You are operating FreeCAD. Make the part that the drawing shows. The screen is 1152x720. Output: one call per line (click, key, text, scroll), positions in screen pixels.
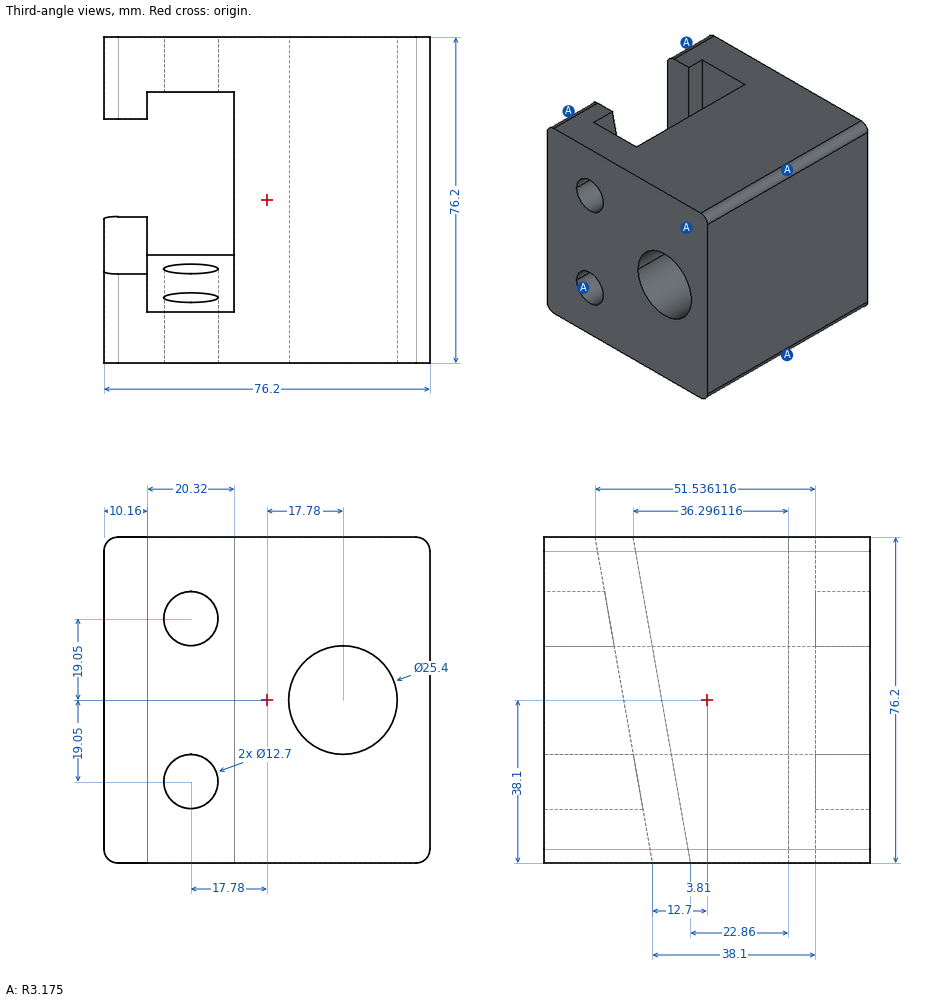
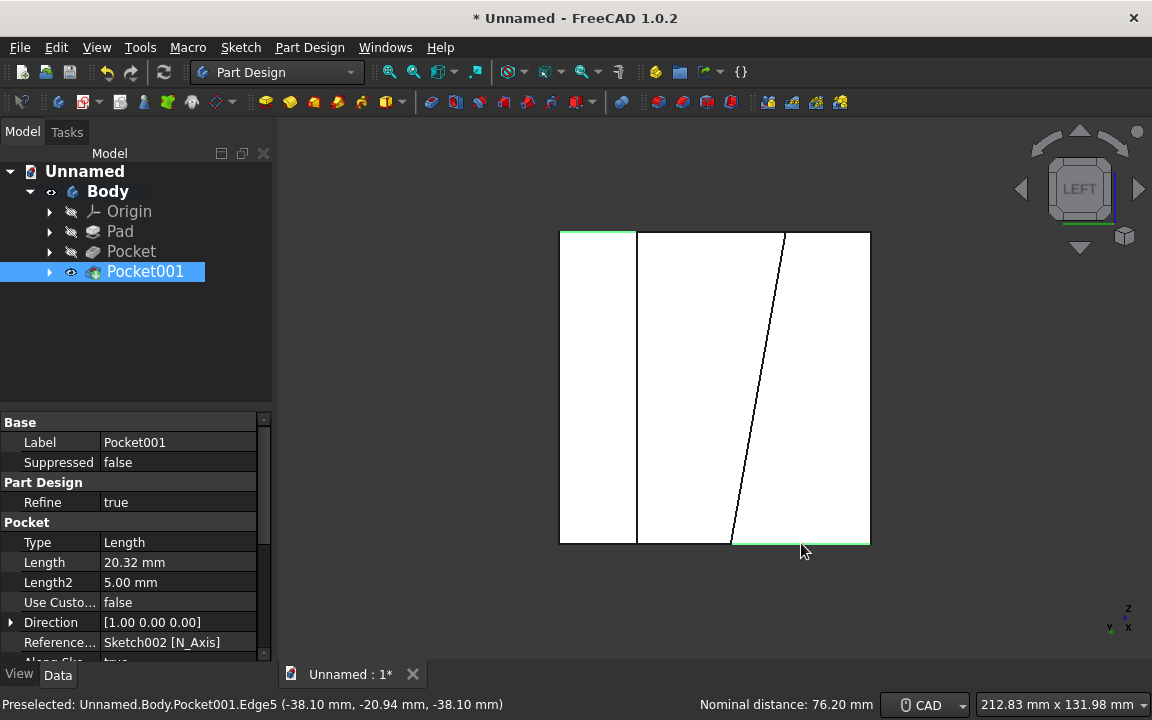
click(829, 231, ctrl)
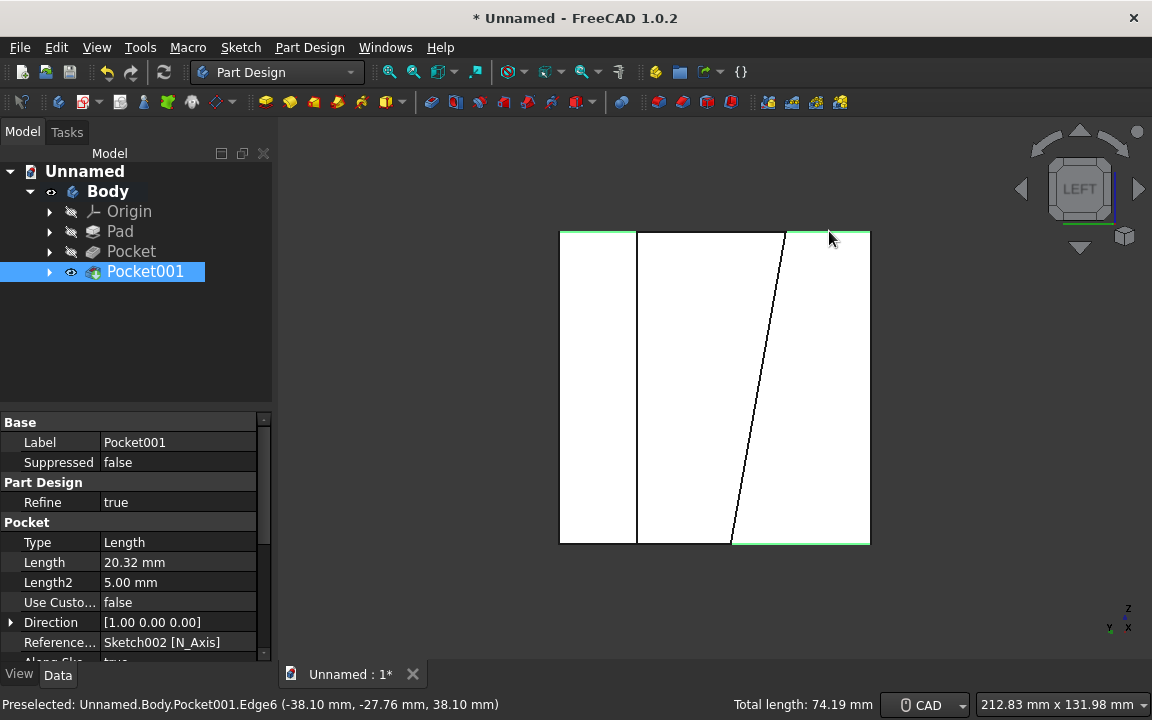
click(598, 543, ctrl)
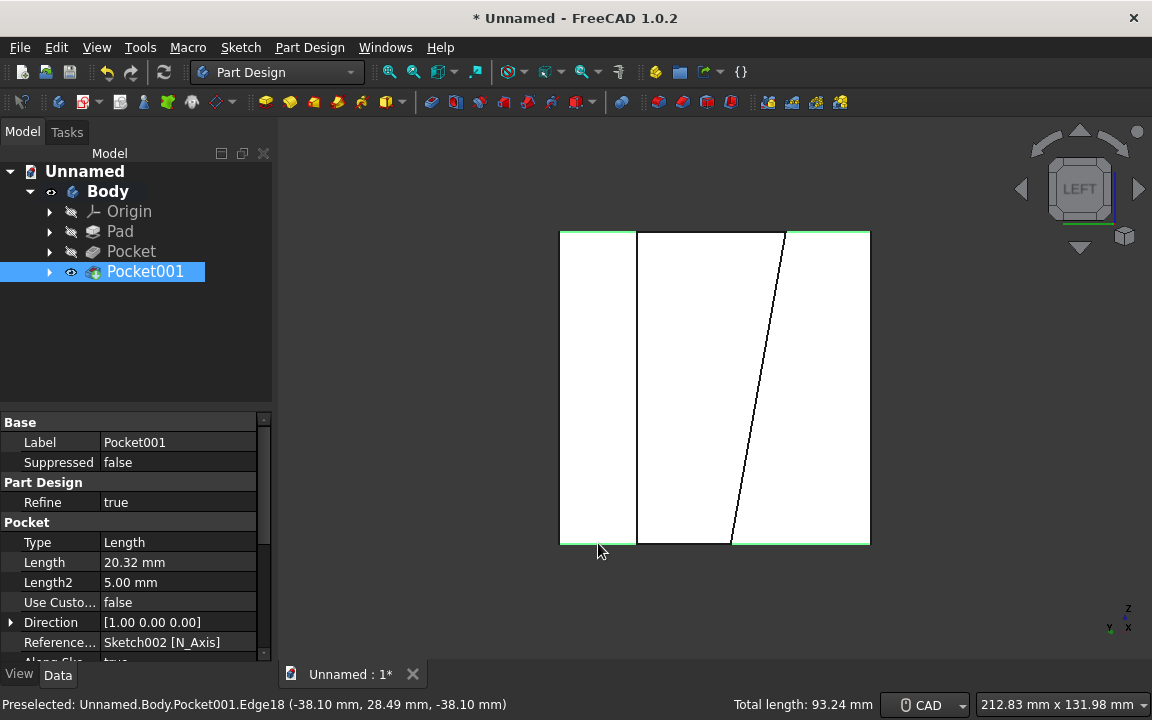
key(0)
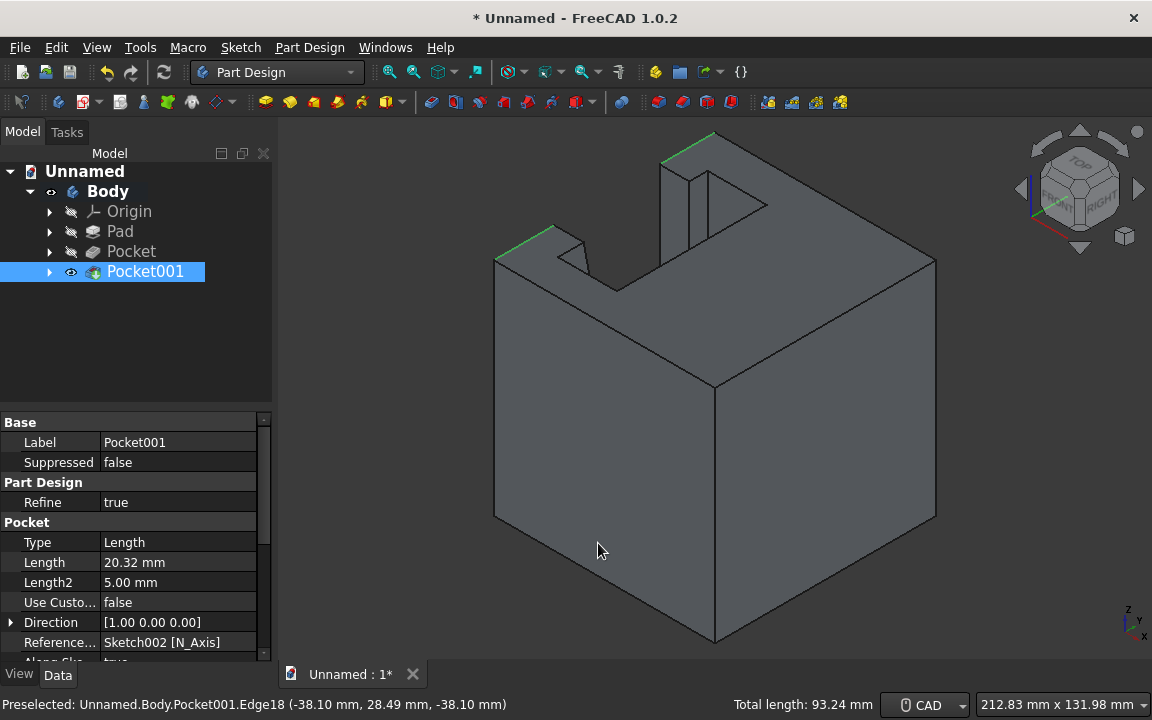
click(826, 323, ctrl)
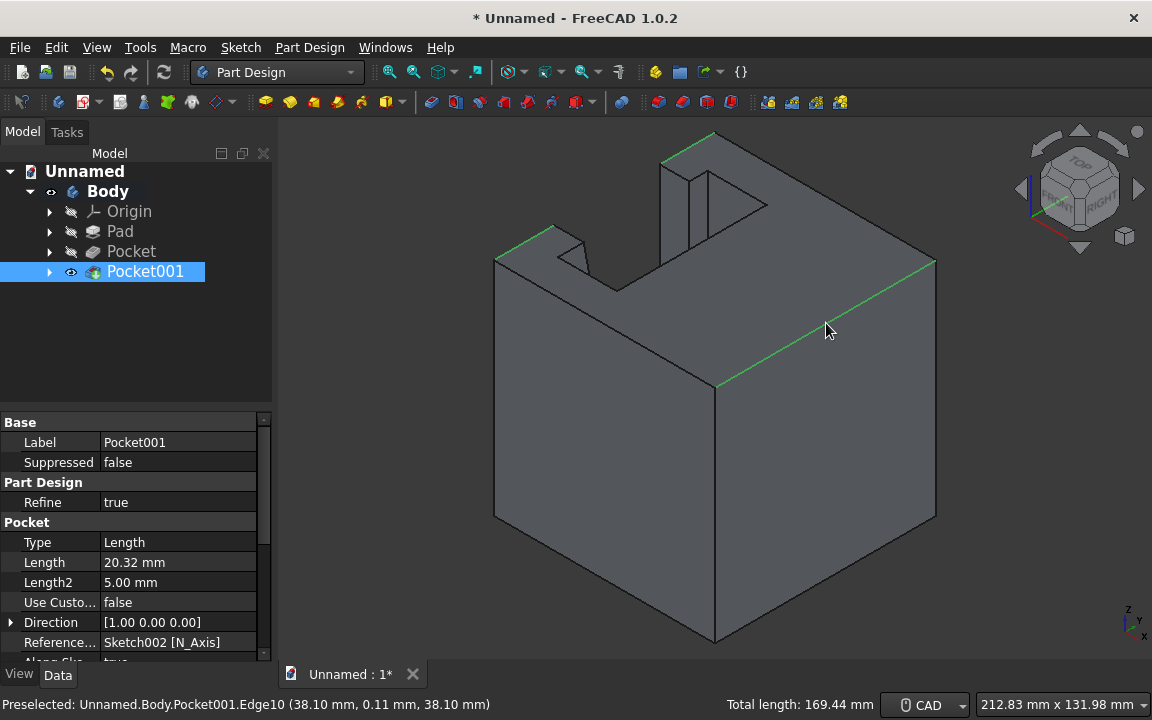
key(2)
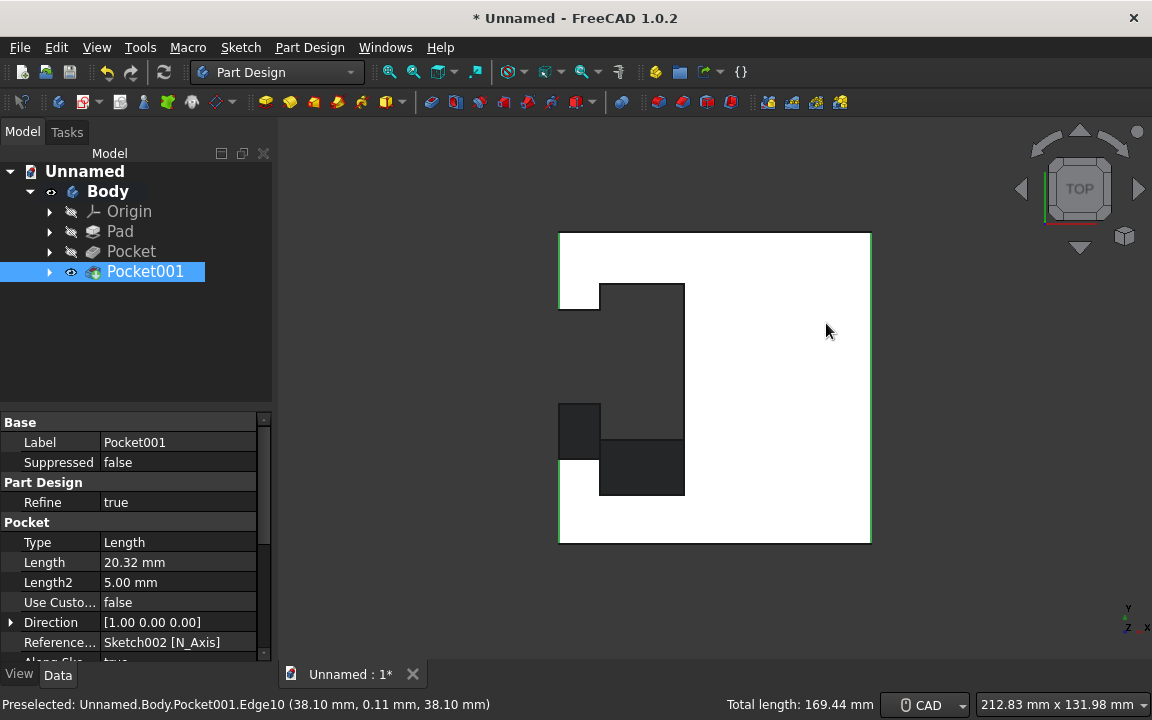
key(1)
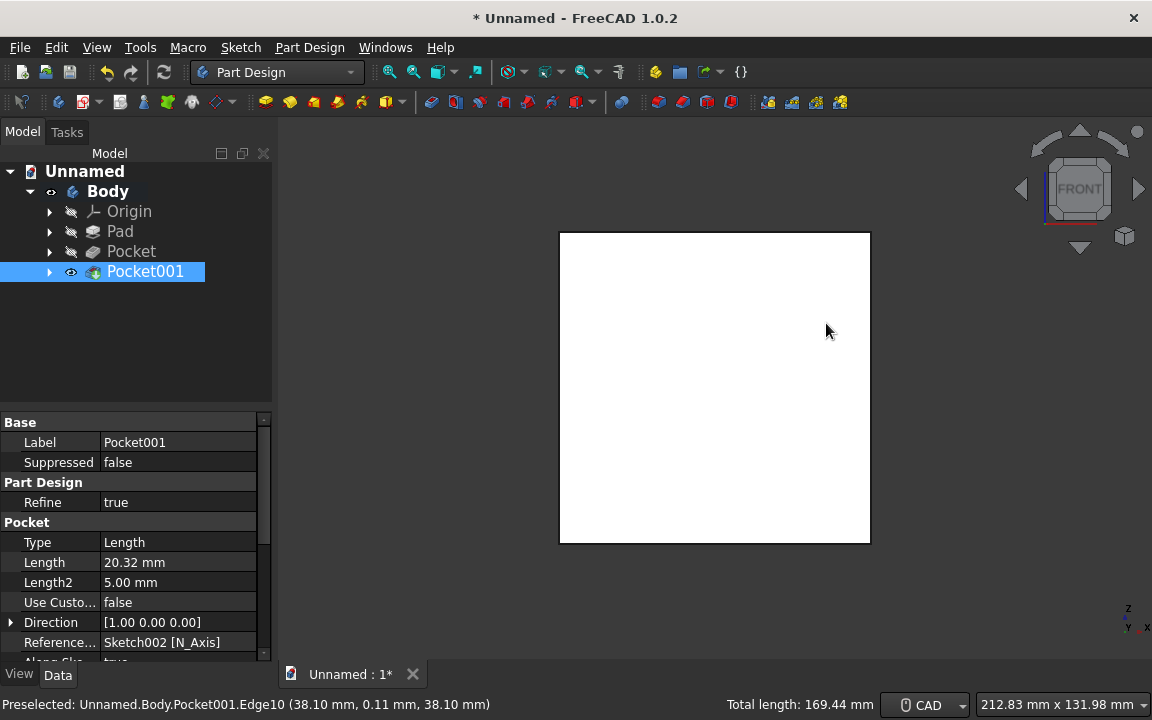
key(3)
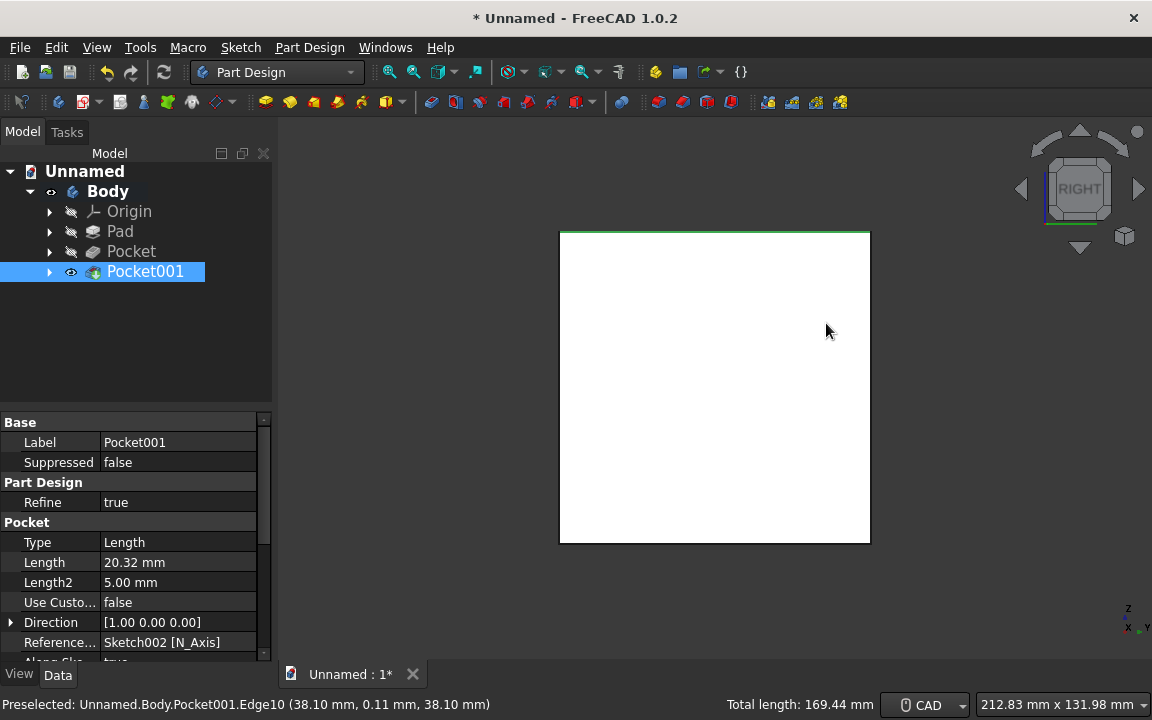
click(715, 543, ctrl)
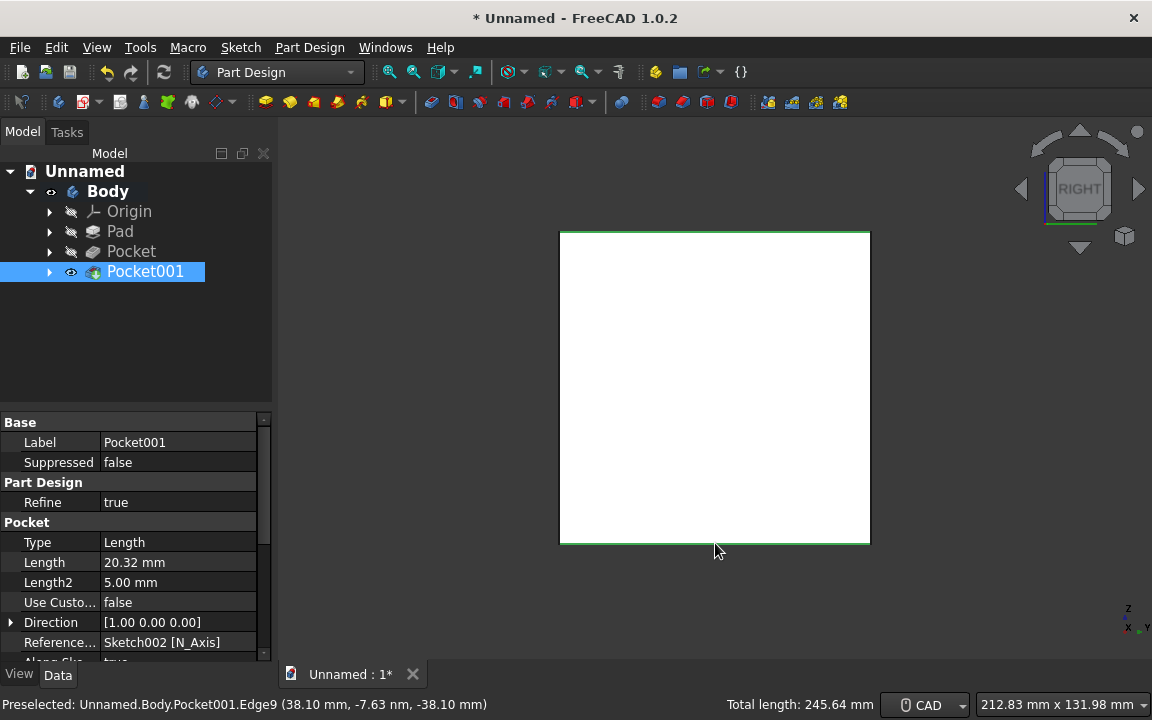
click(660, 102)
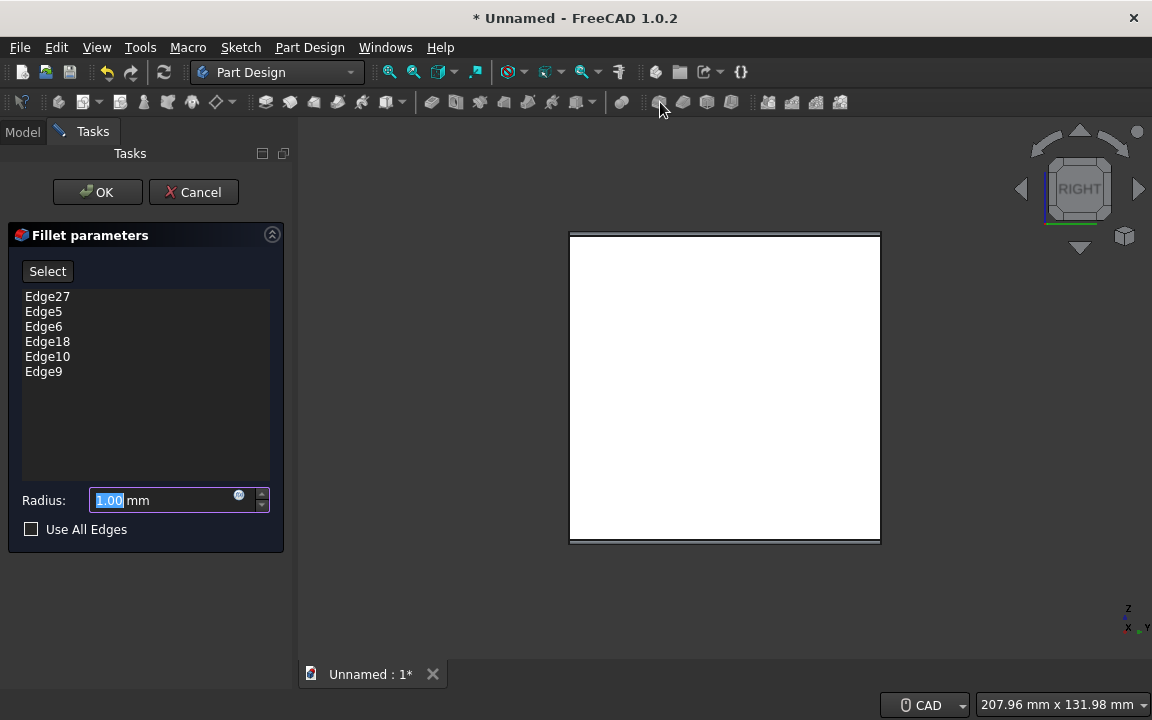
text(3.175)
key(Tab)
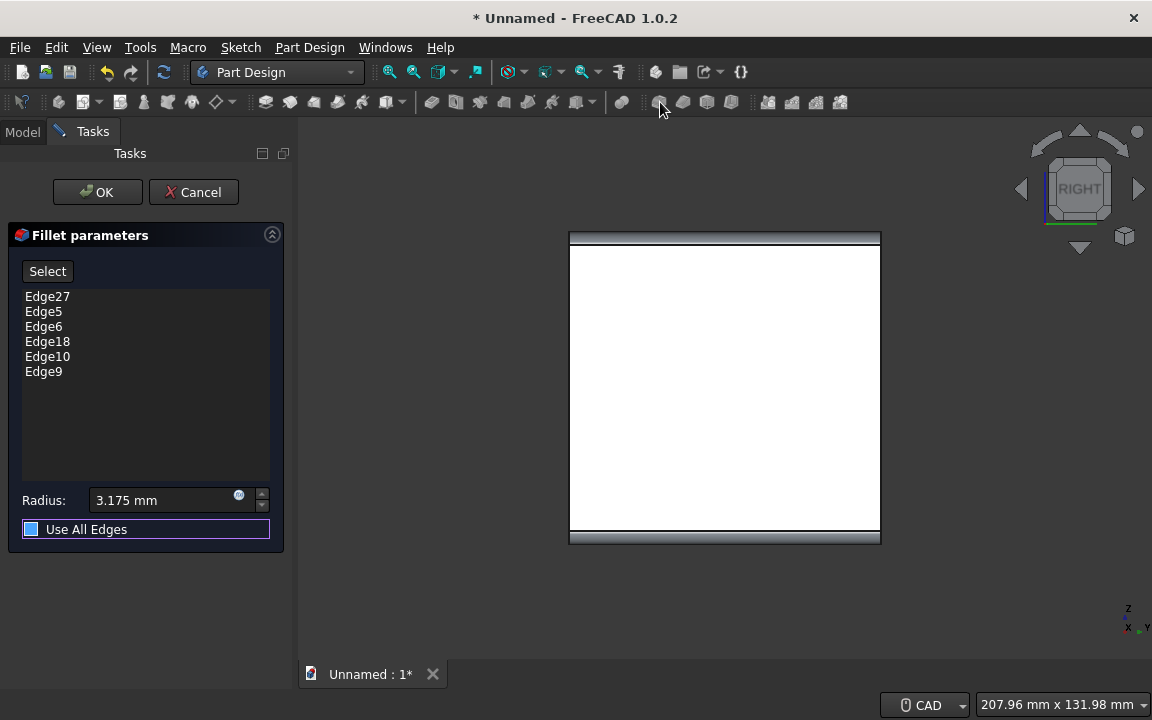
click(98, 192)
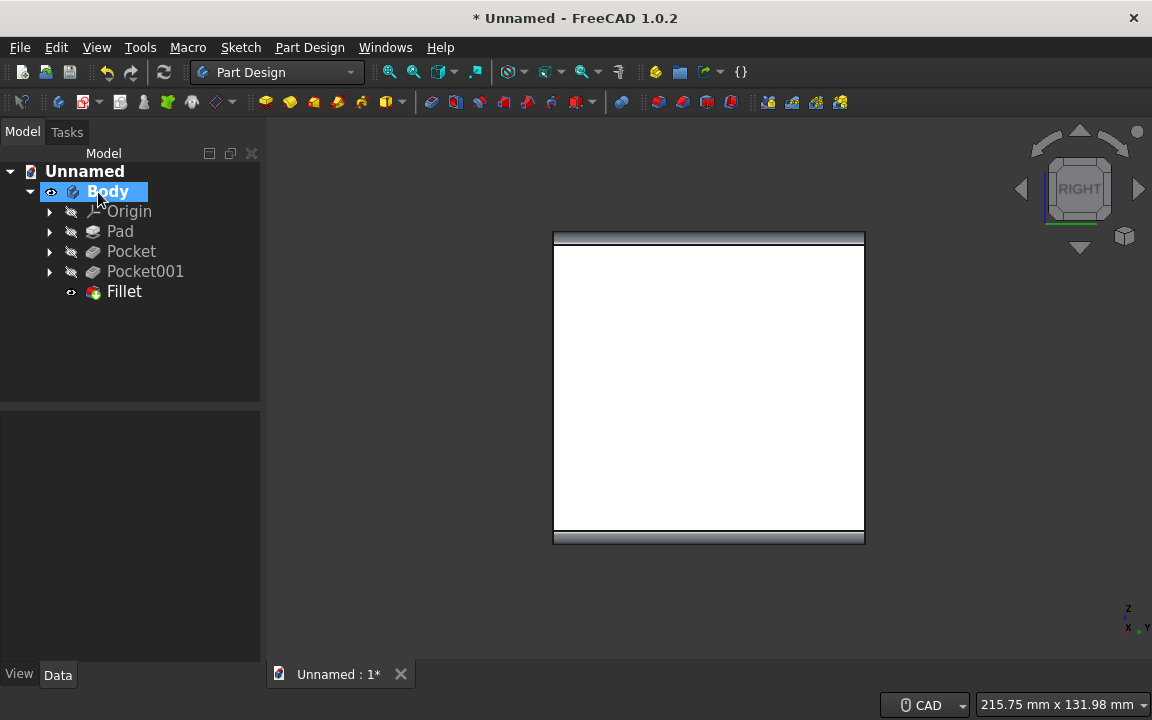
key(4)